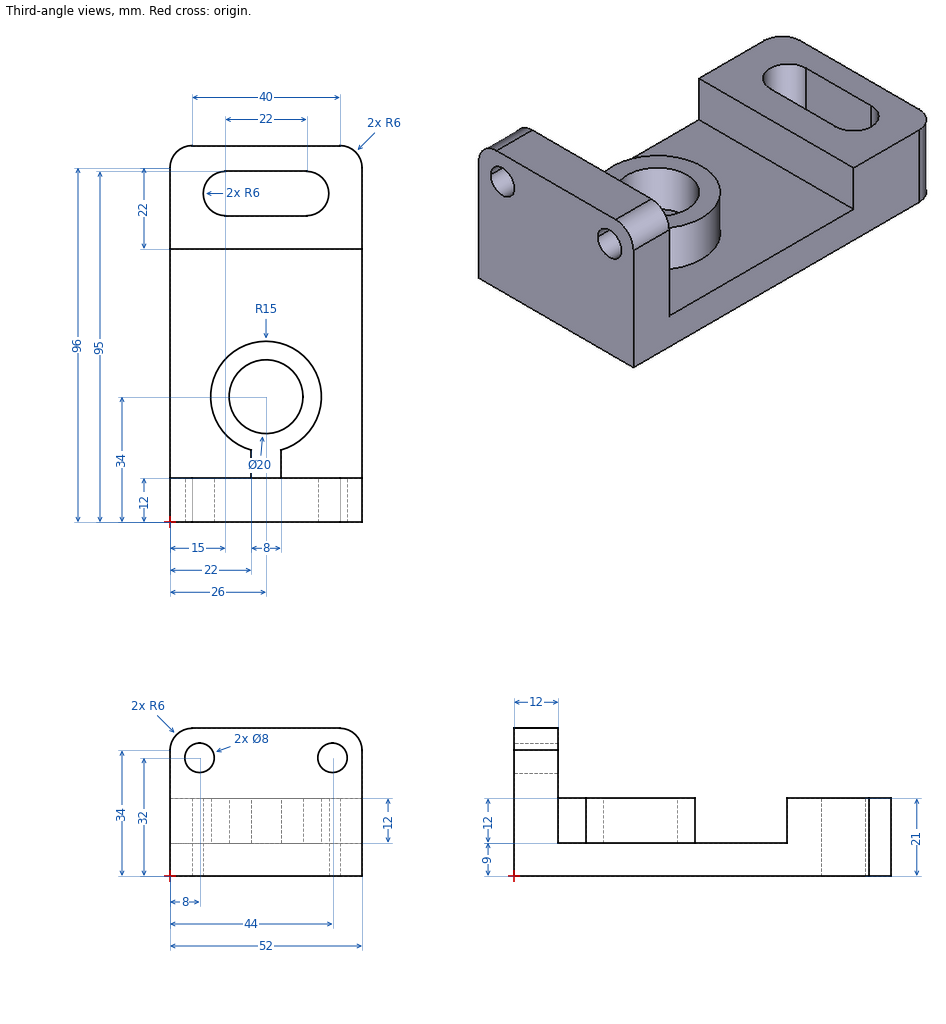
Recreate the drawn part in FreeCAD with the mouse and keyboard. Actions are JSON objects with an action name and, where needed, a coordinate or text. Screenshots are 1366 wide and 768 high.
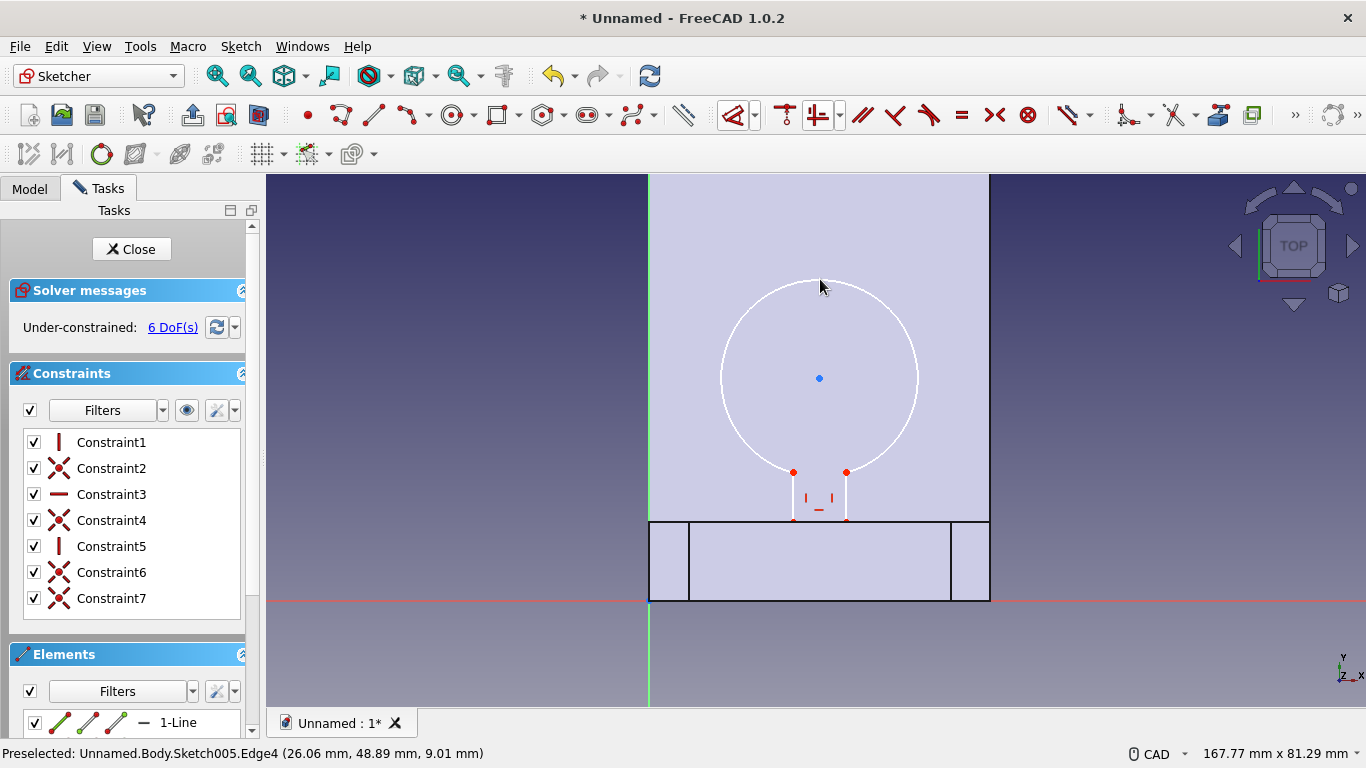
{"action": "left_click", "coordinate": [909, 338]}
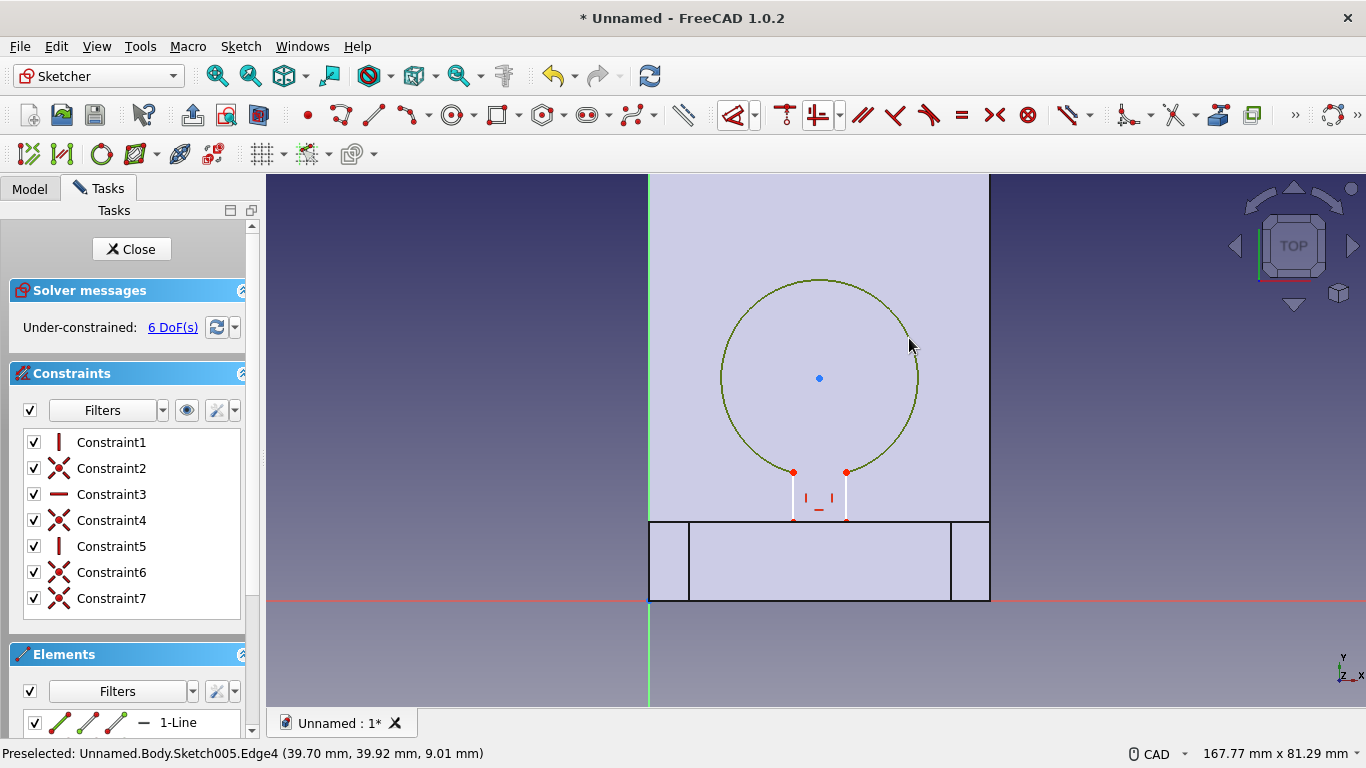
{"action": "key", "text": "k r"}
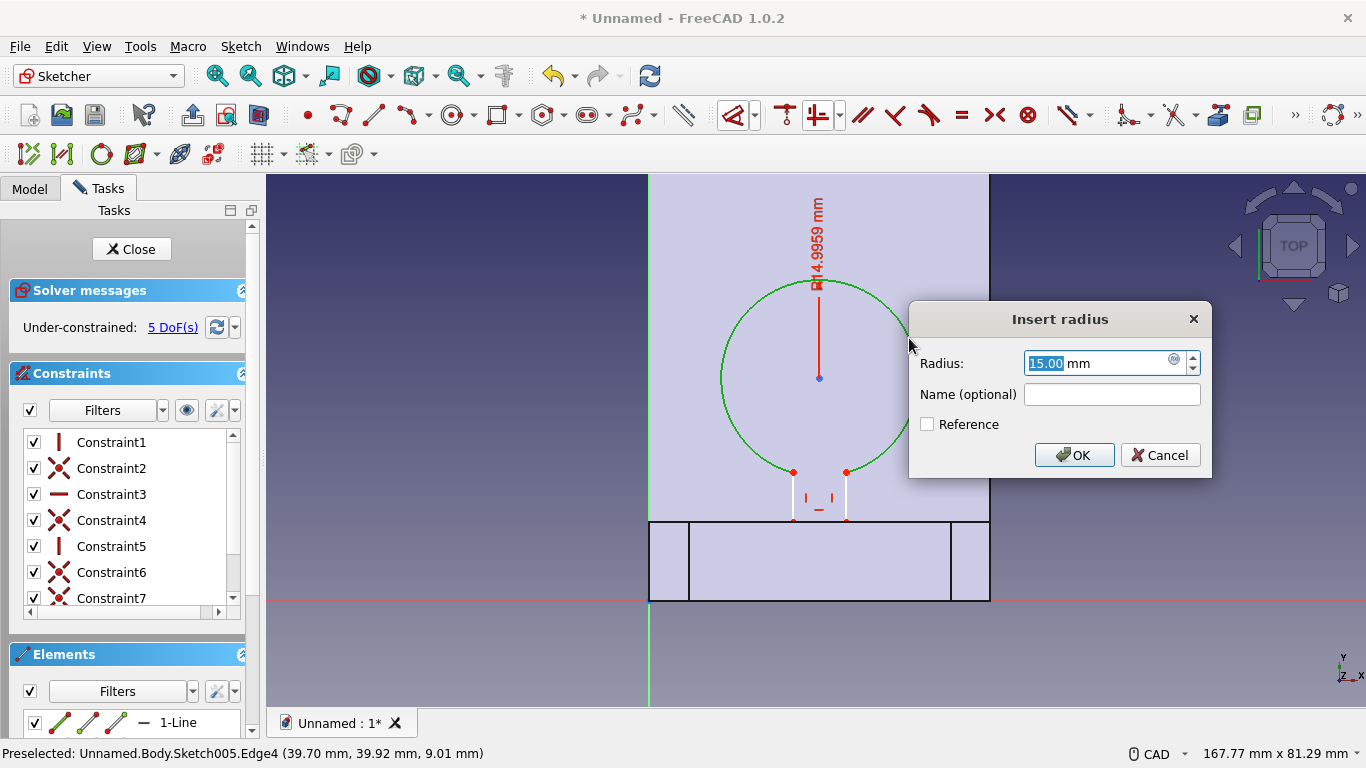
{"action": "type", "text": "15"}
{"action": "key", "text": "Return"}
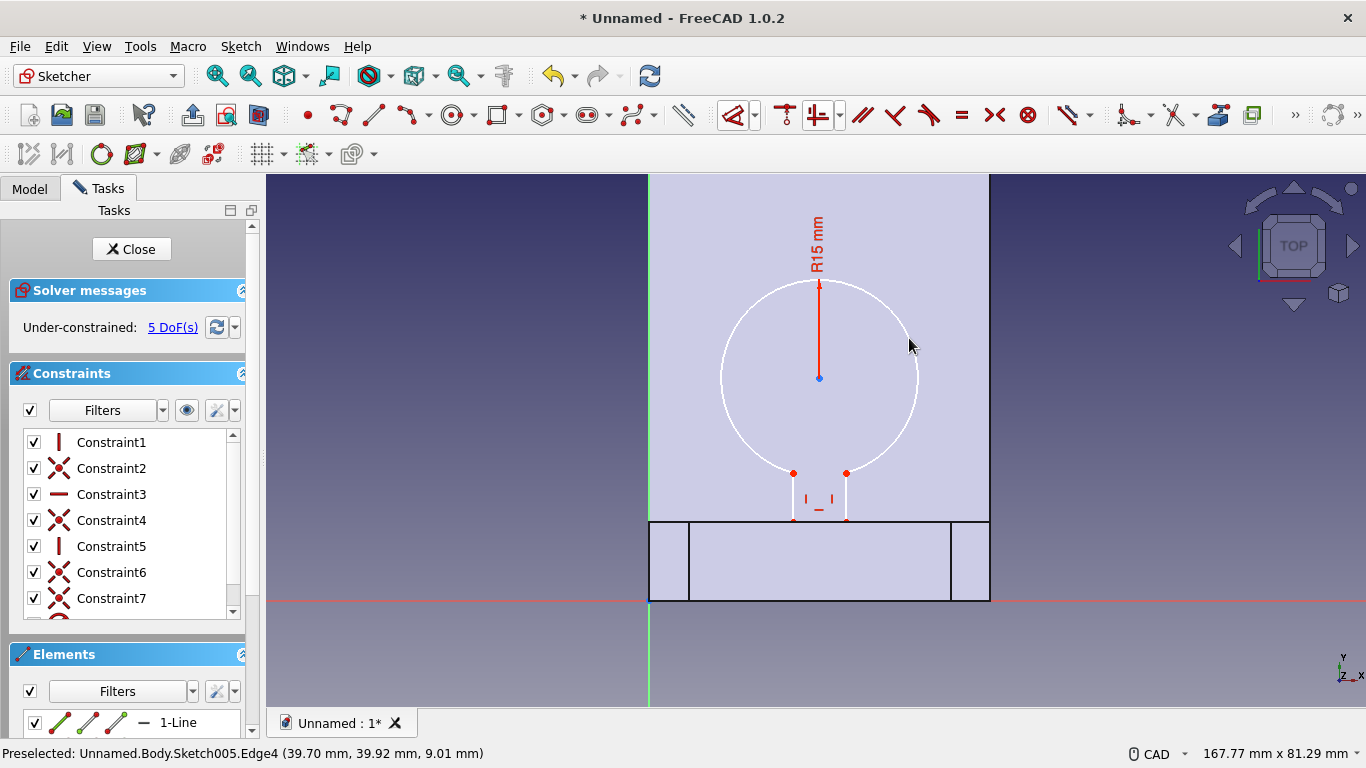
{"action": "left_click", "coordinate": [809, 523]}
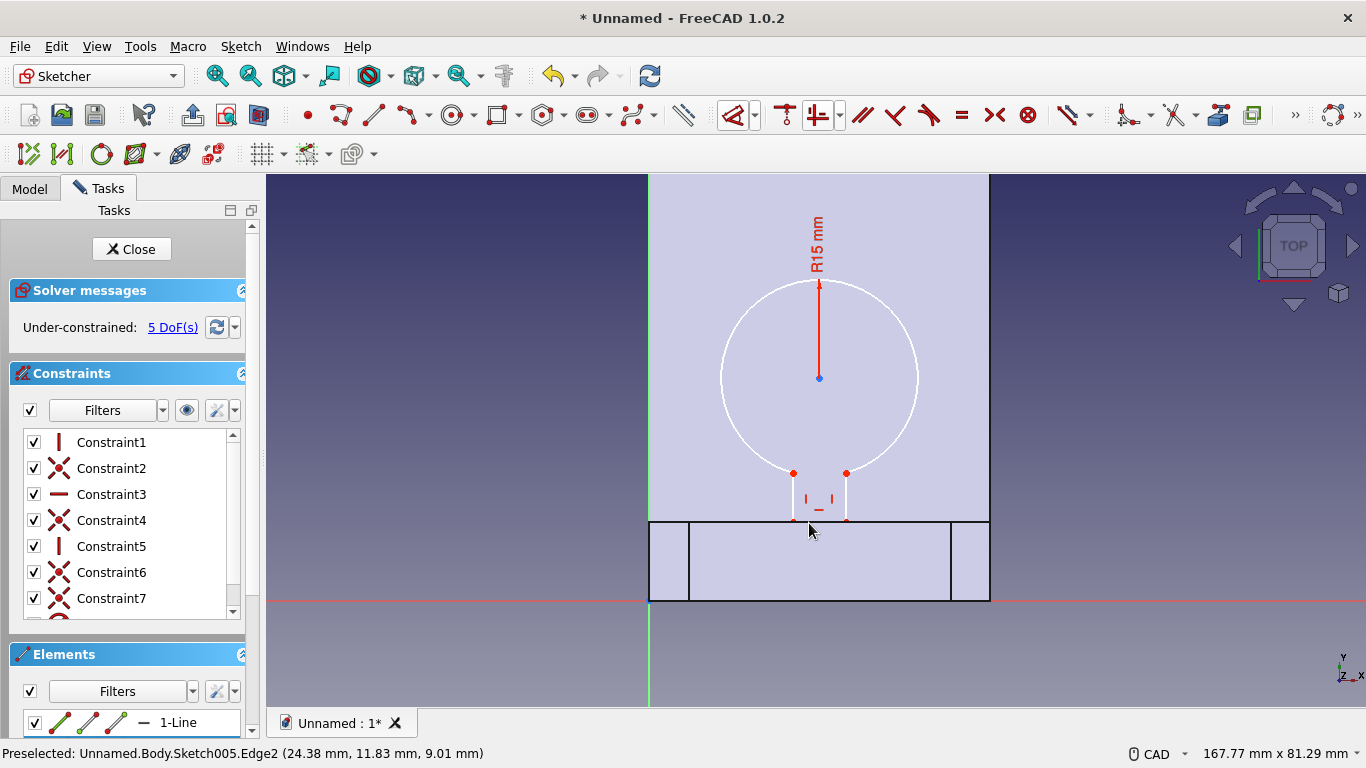
{"action": "left_click", "coordinate": [754, 116]}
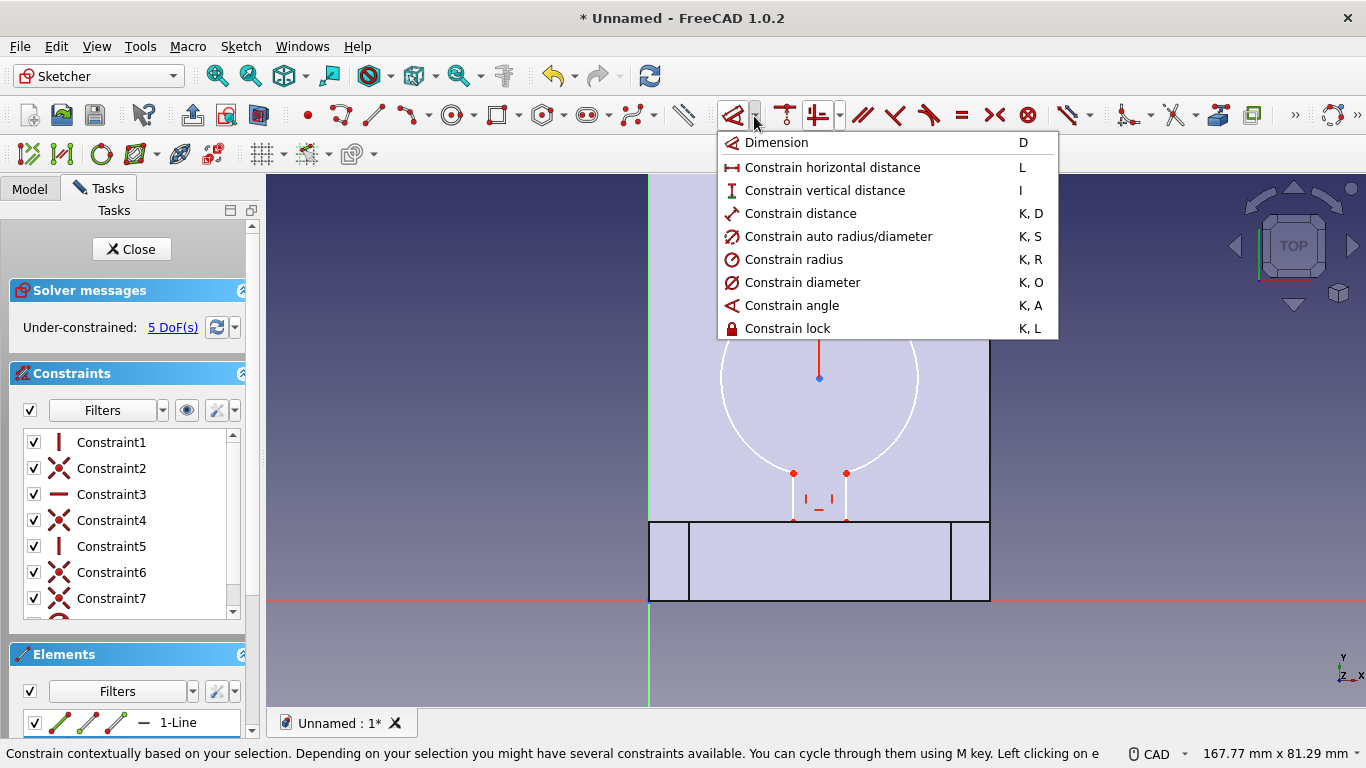
{"action": "left_click", "coordinate": [888, 168]}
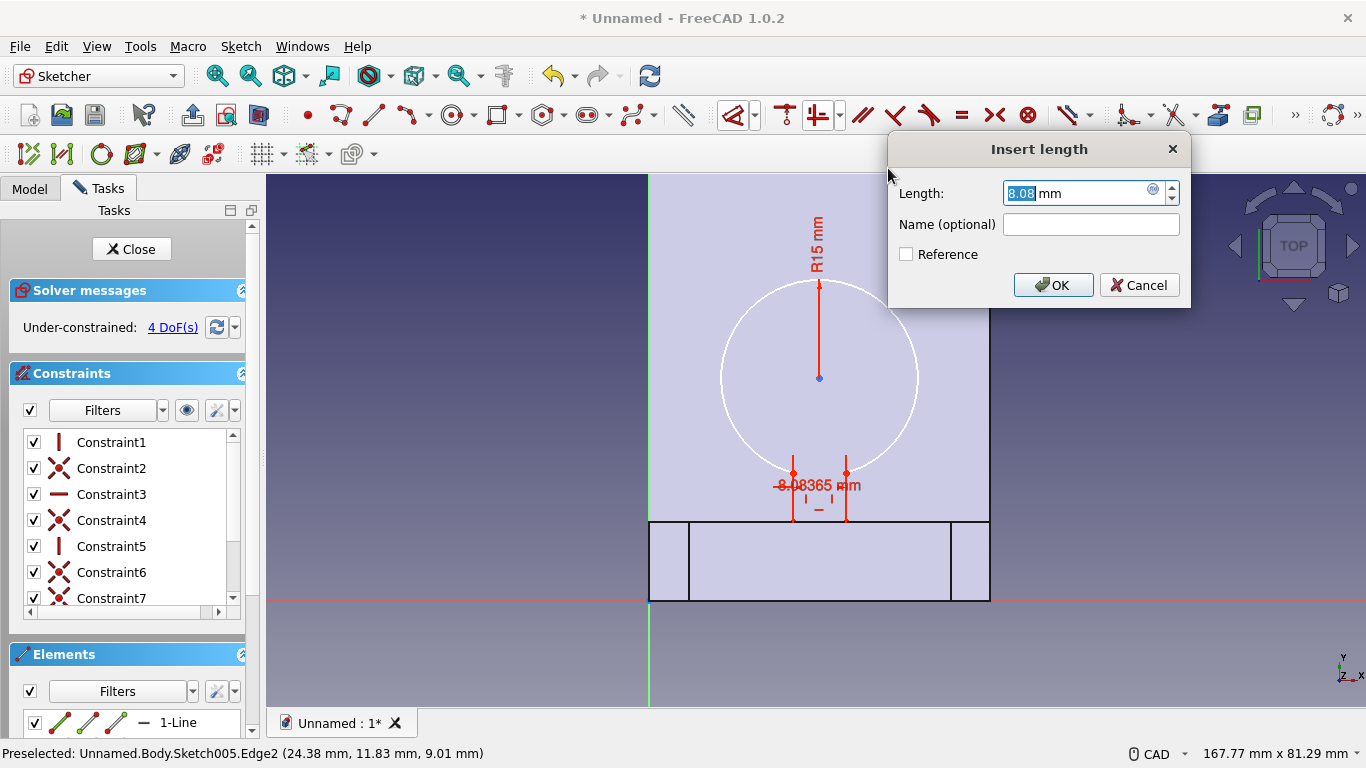
{"action": "type", "text": "8"}
{"action": "key", "text": "Return"}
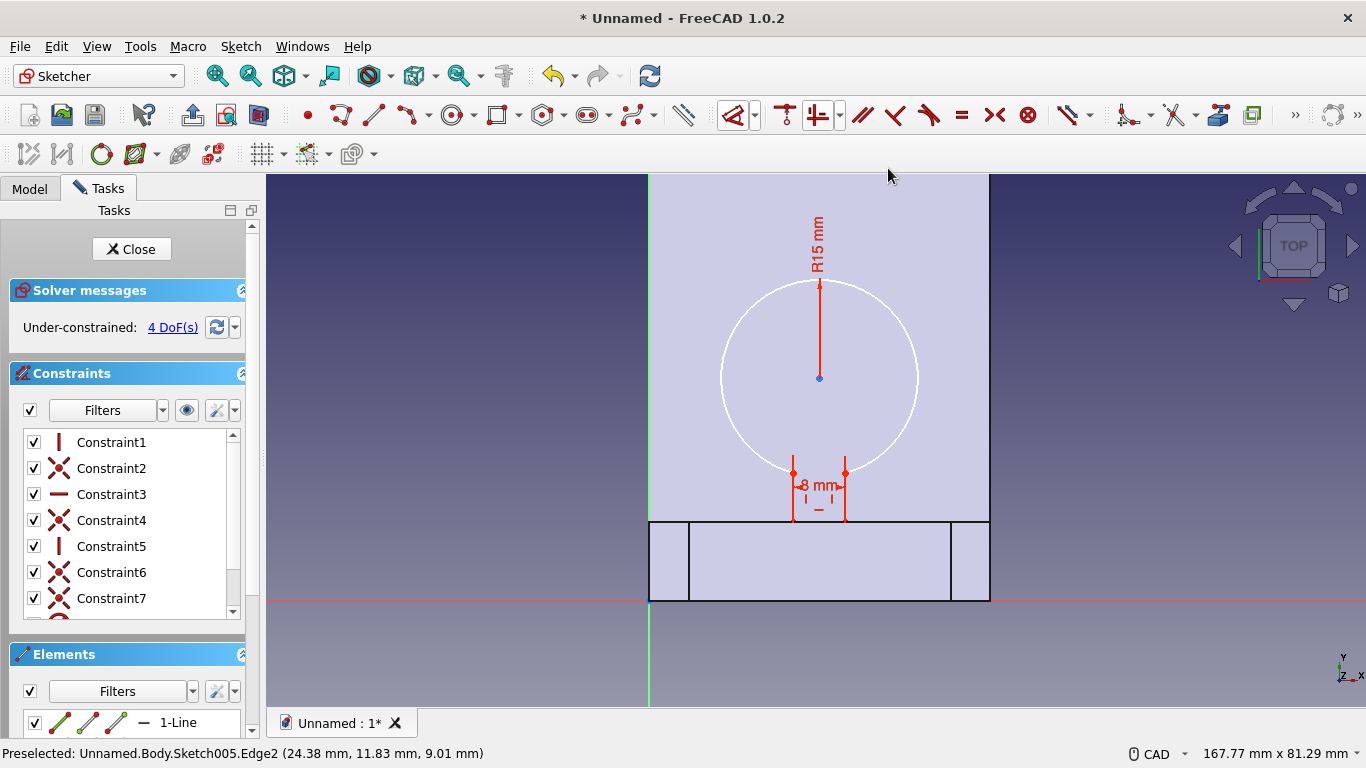
{"action": "left_click", "coordinate": [793, 473]}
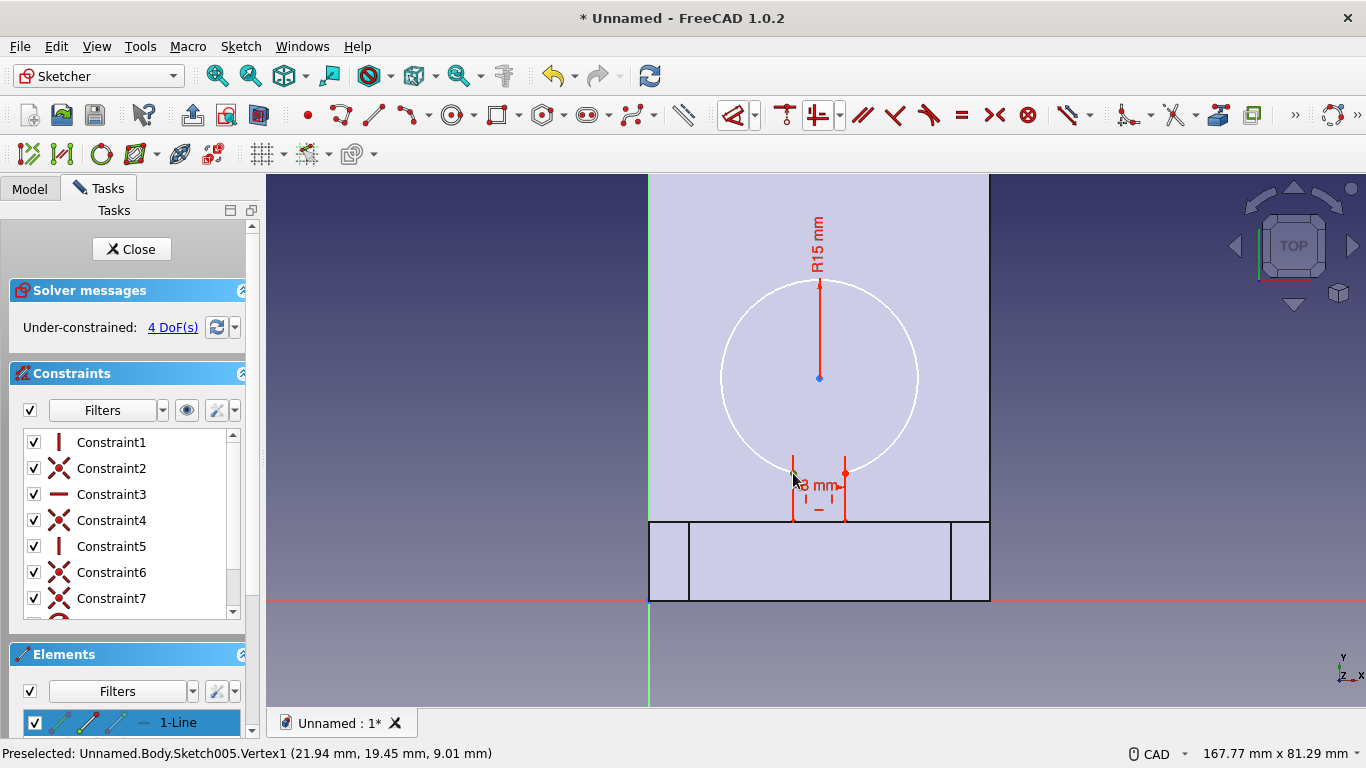
{"action": "key", "text": "l"}